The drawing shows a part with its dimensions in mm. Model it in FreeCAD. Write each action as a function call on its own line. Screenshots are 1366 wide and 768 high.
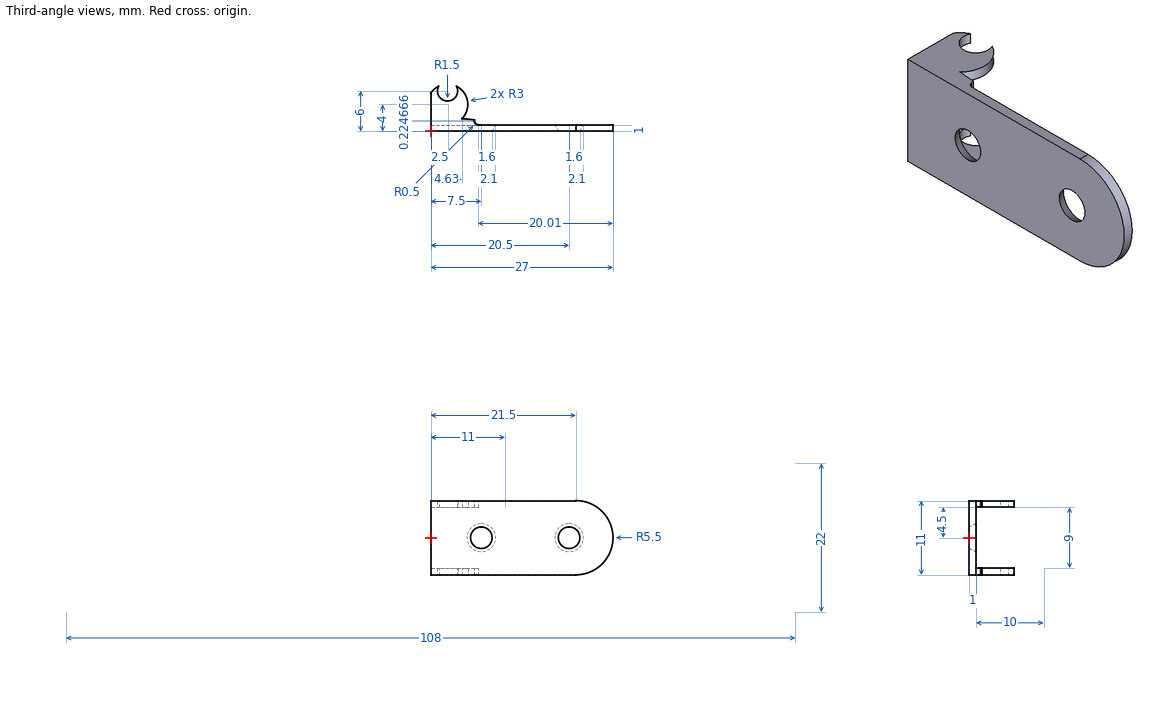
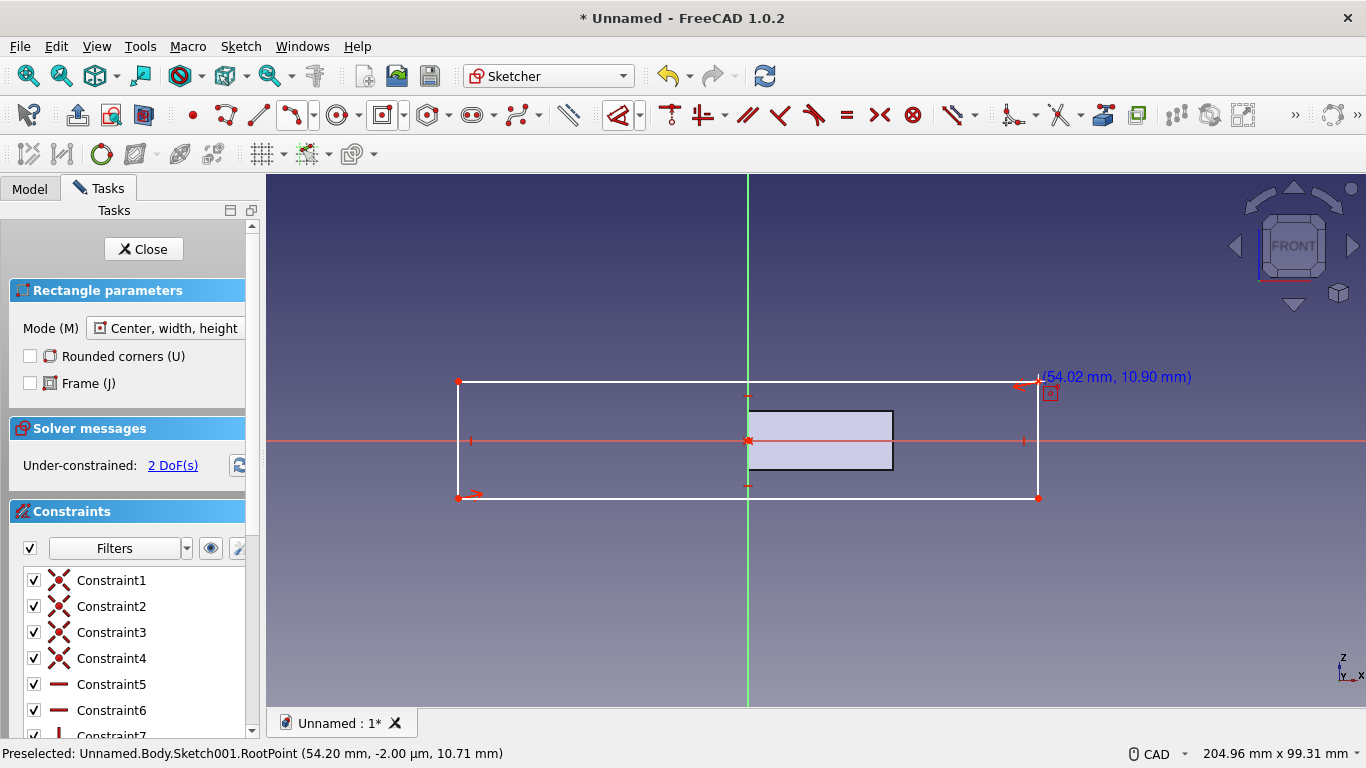
click(226, 116)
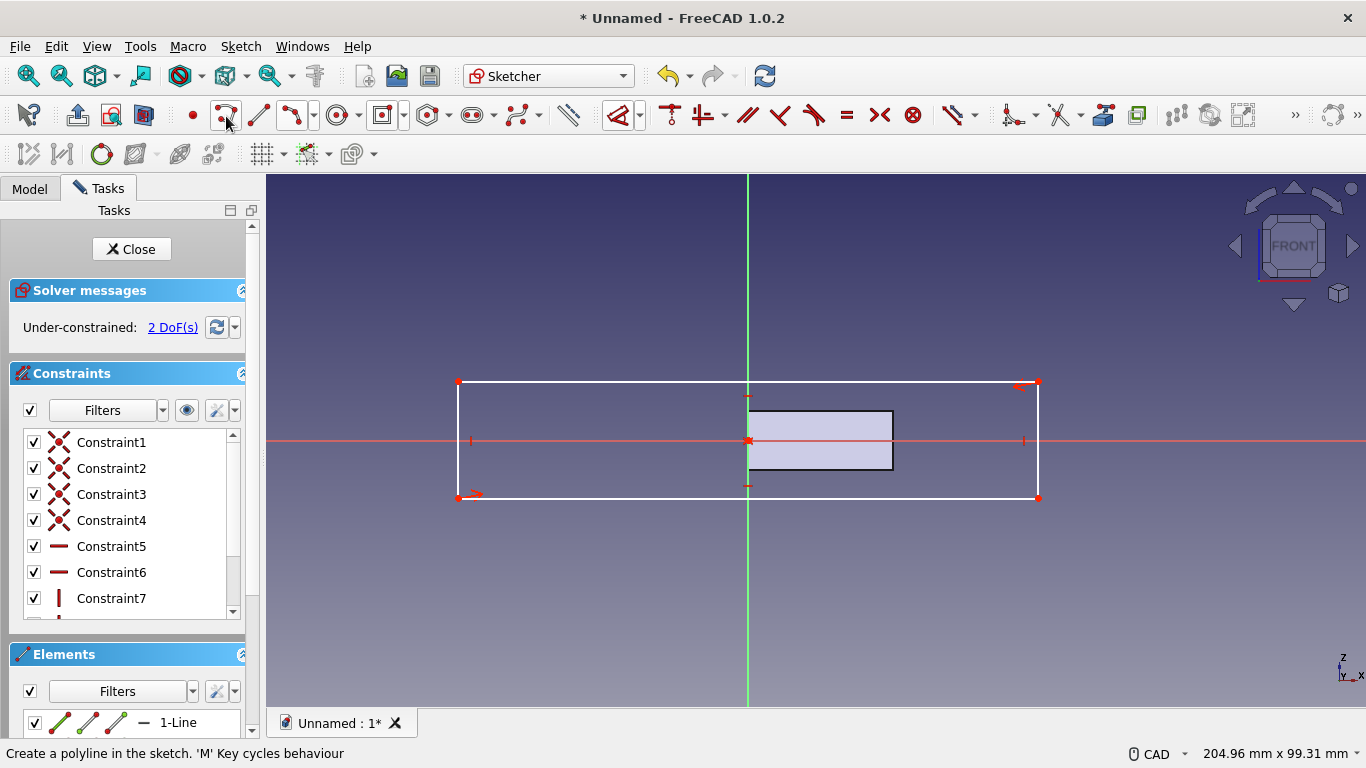
click(863, 411)
click(748, 411)
click(757, 470)
click(863, 470)
right_click(863, 470)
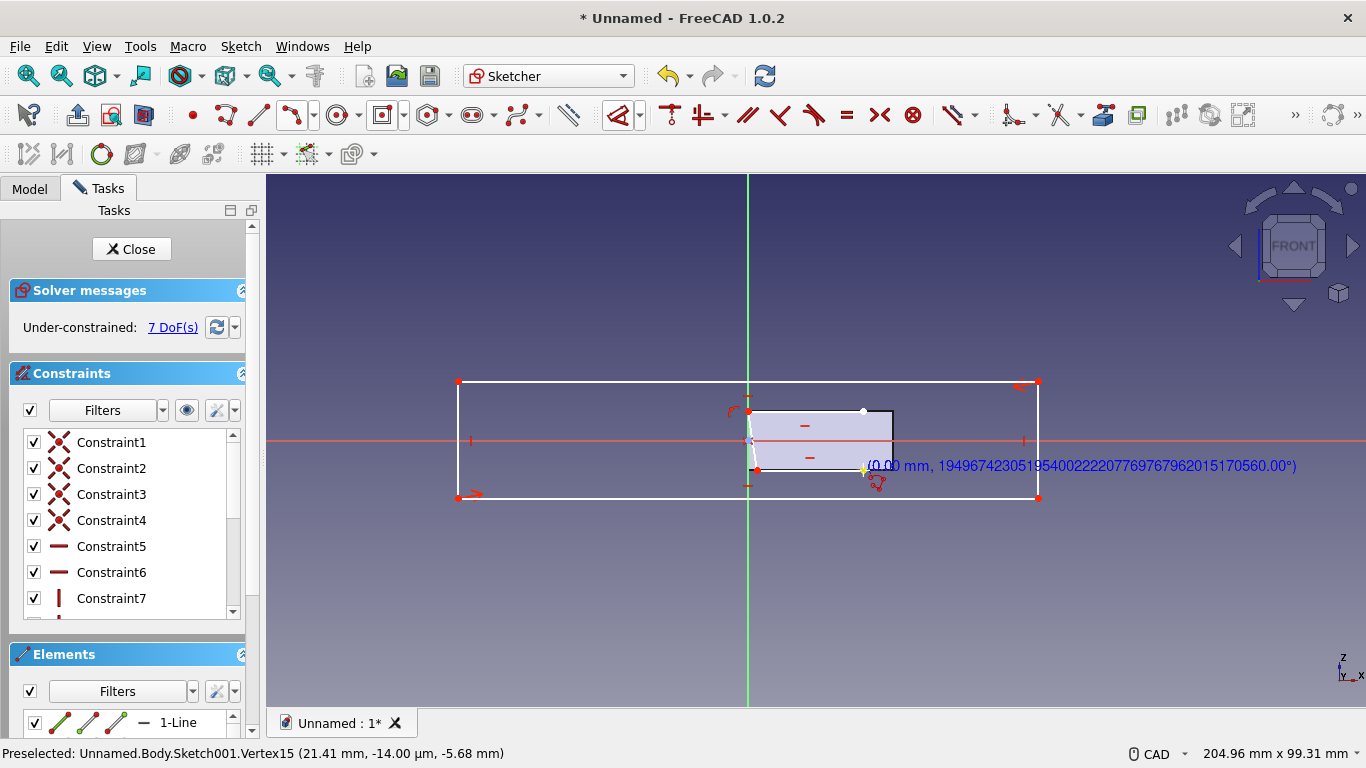
key(g)
key(3)
key(a)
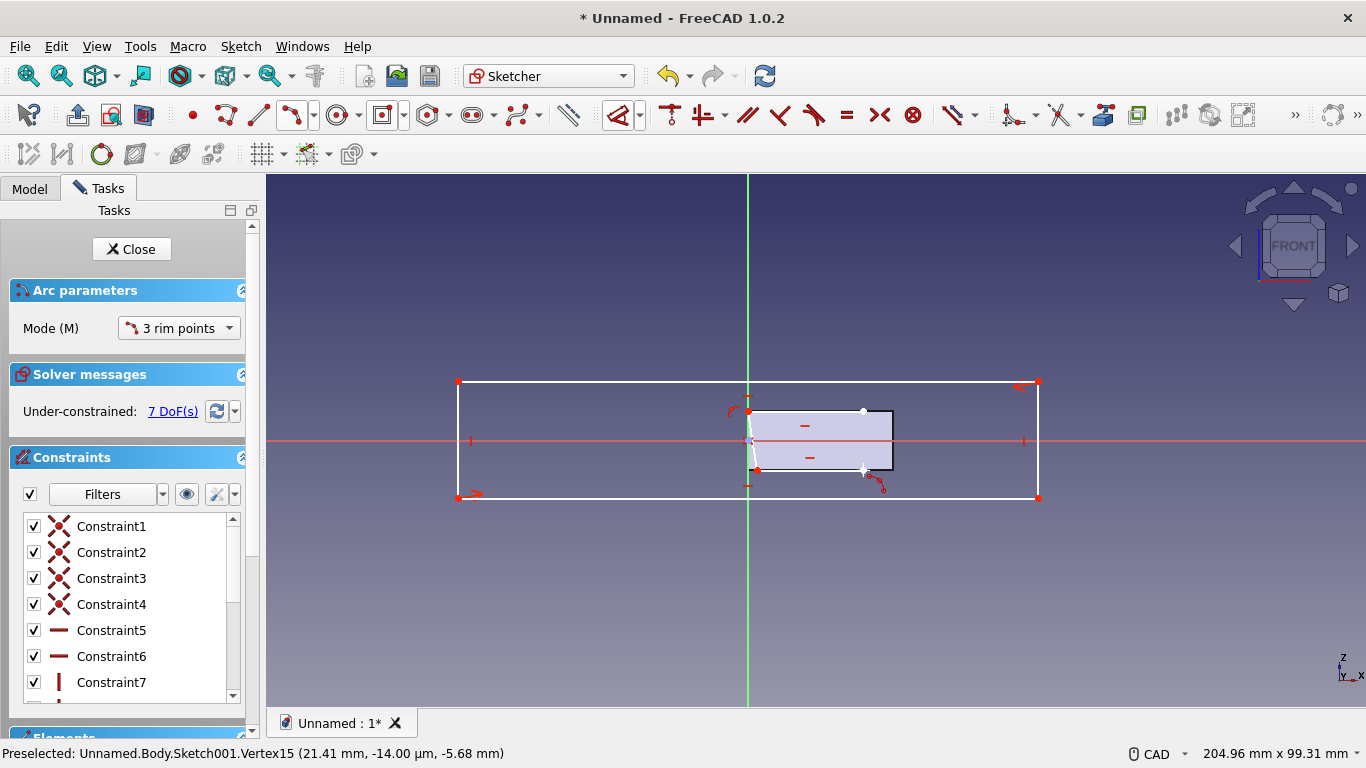
click(863, 471)
click(863, 412)
click(887, 458)
key(Escape)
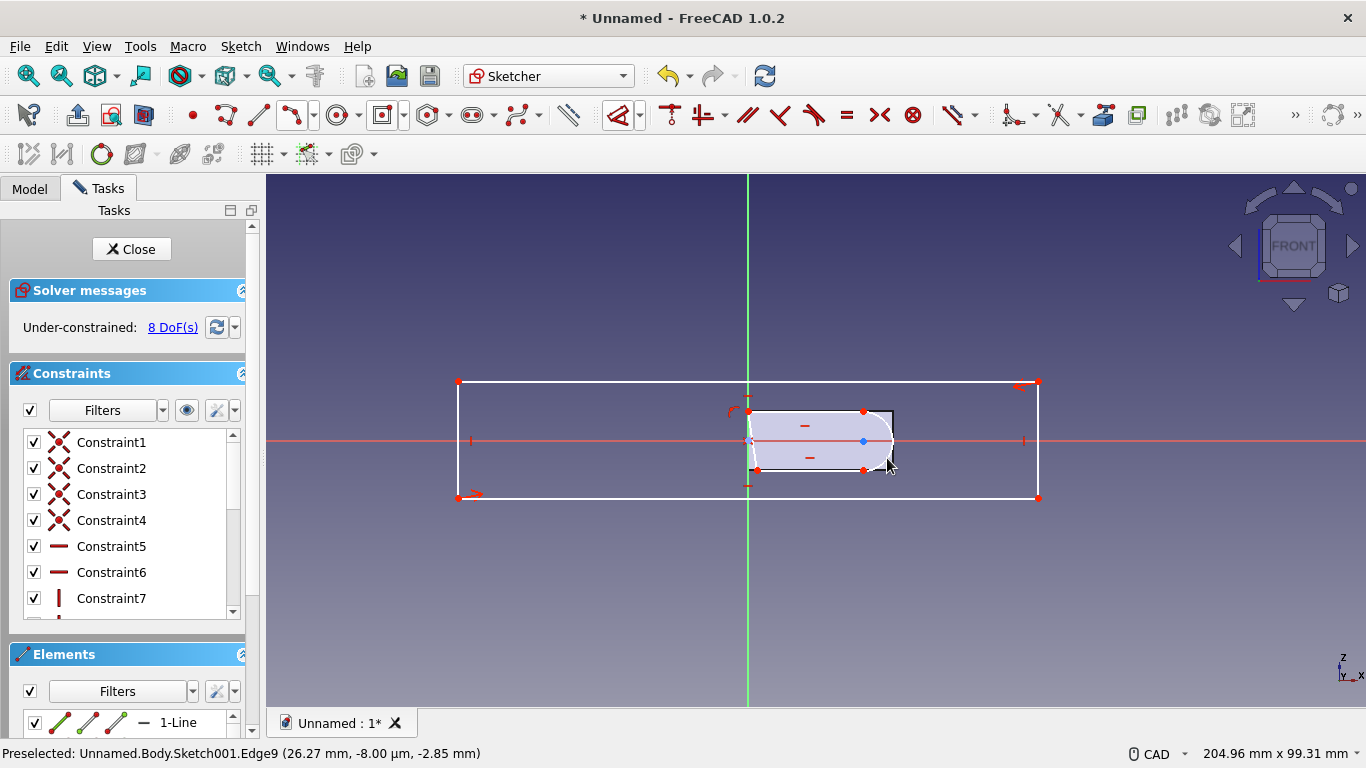
click(829, 412)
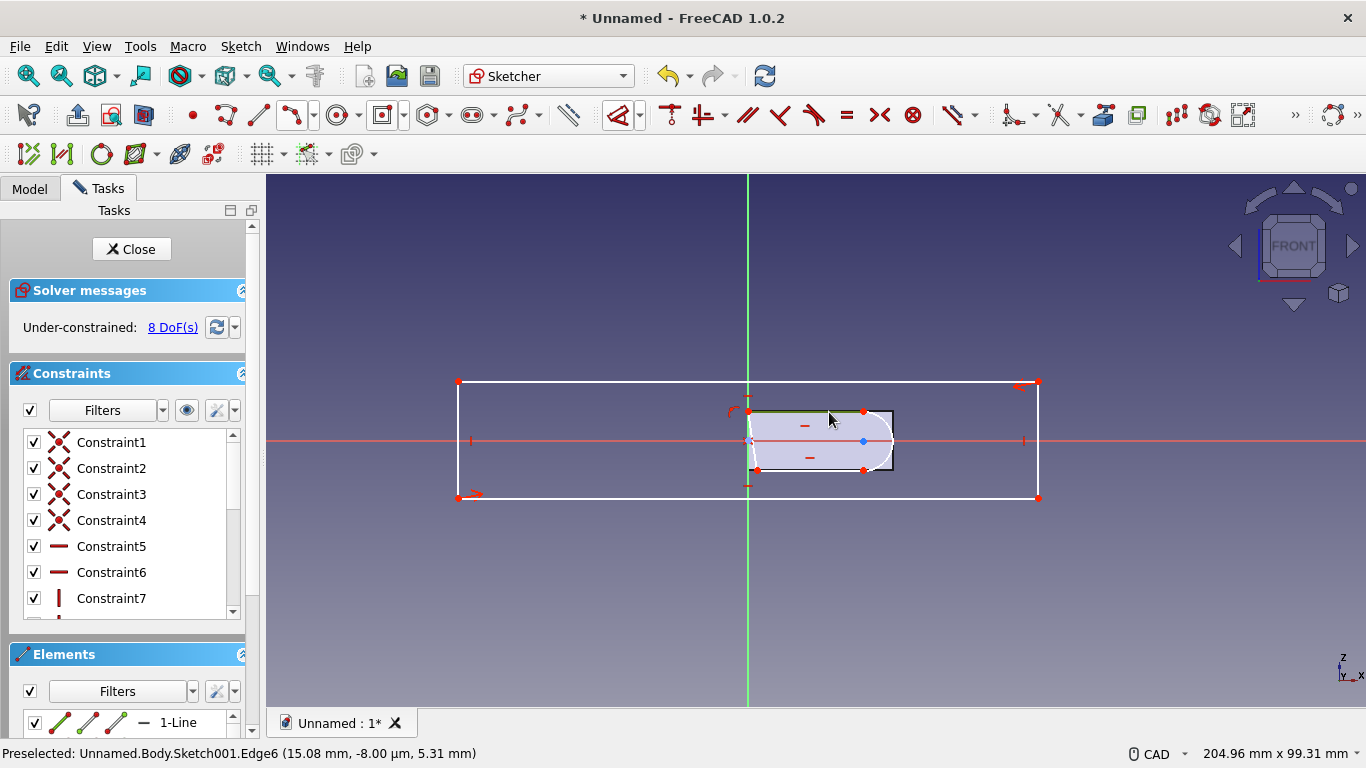
click(887, 459)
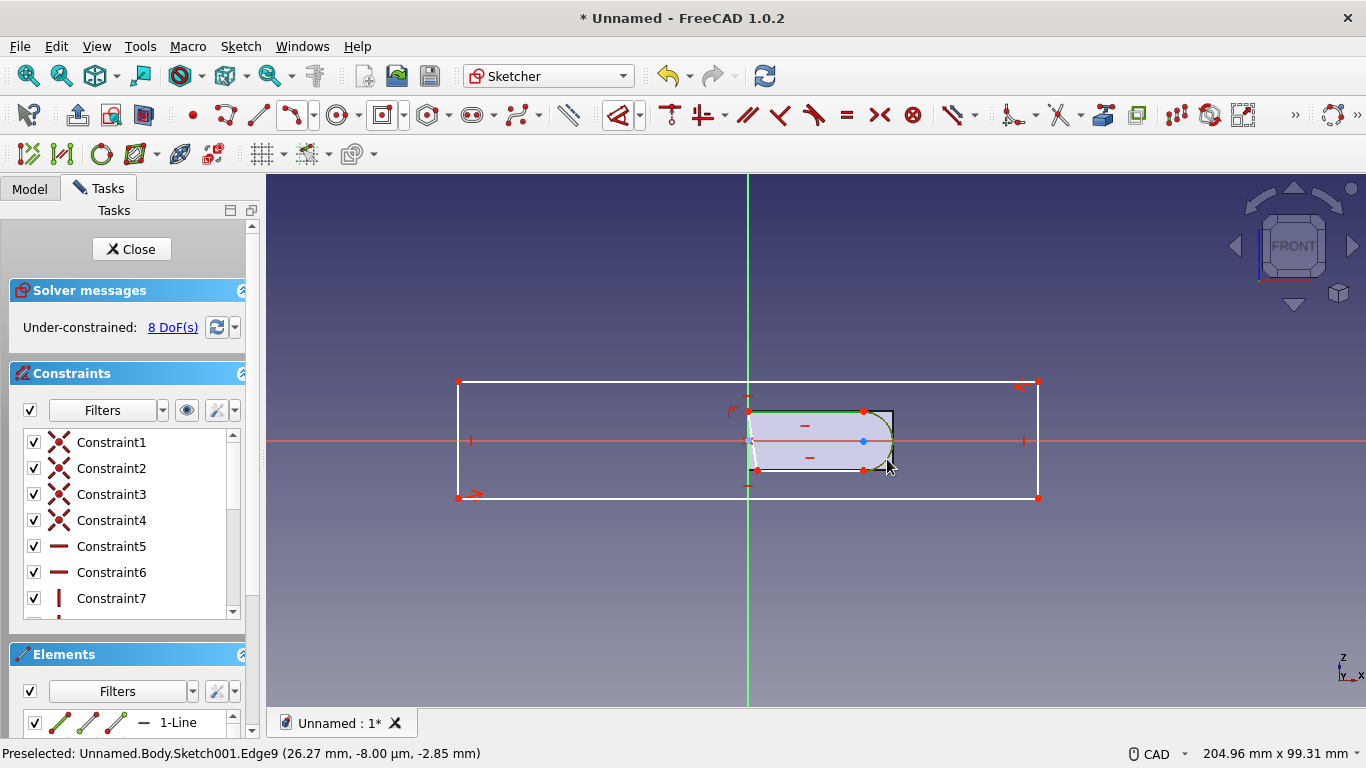
key(t)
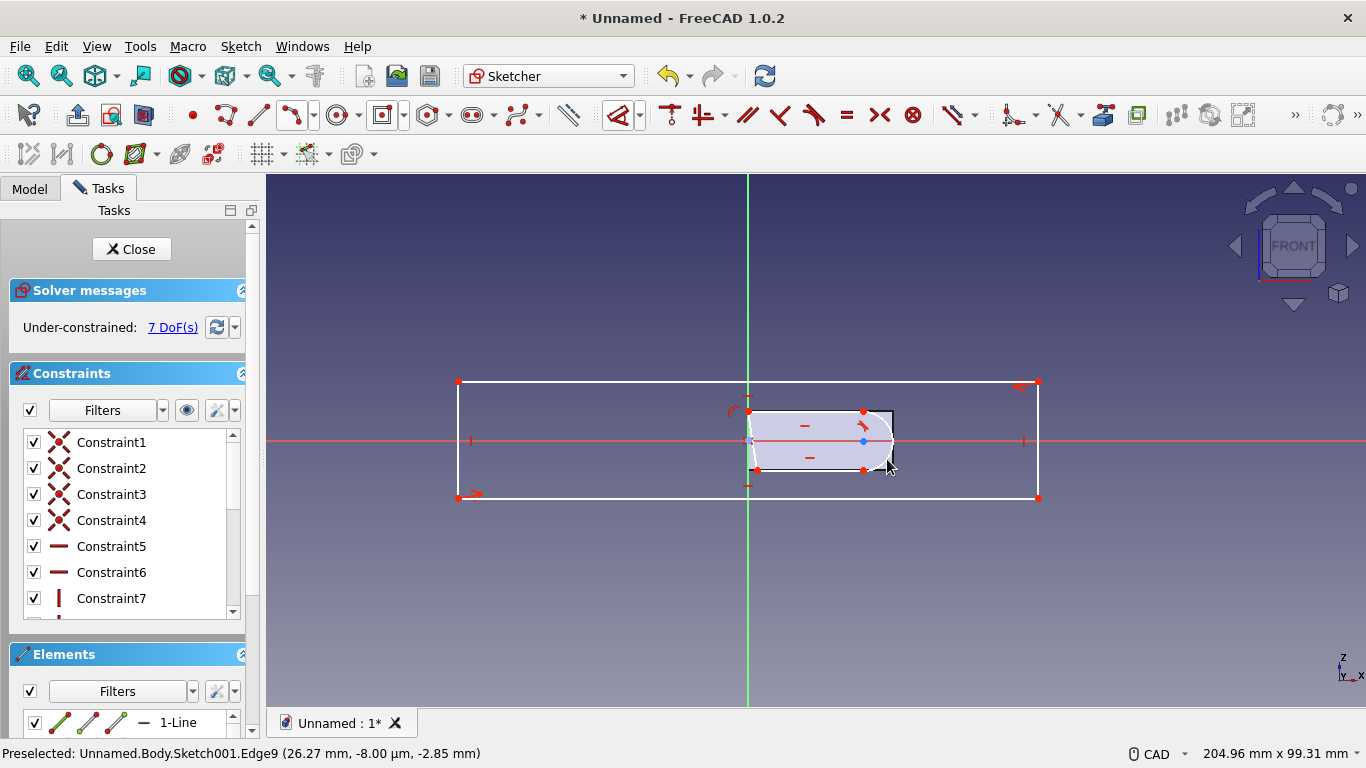
click(789, 471)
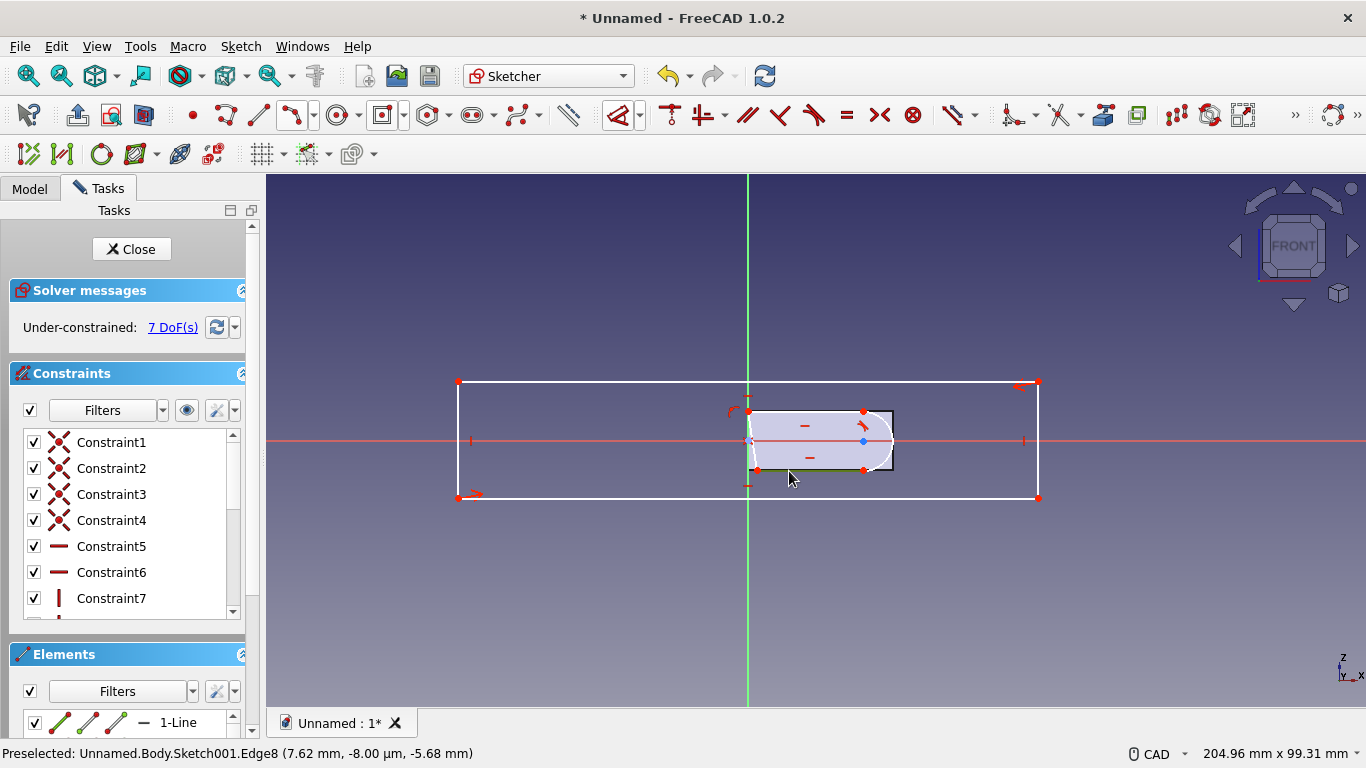
click(887, 459)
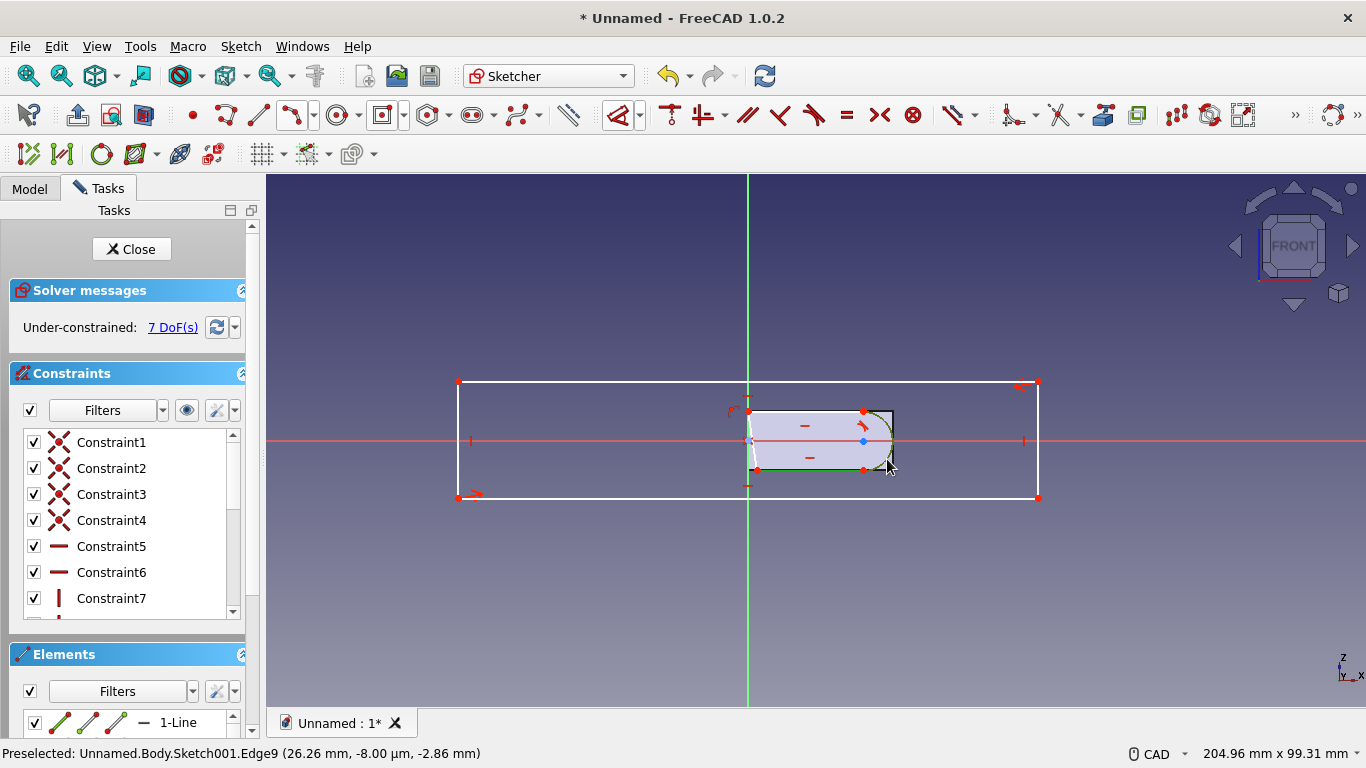
key(t)